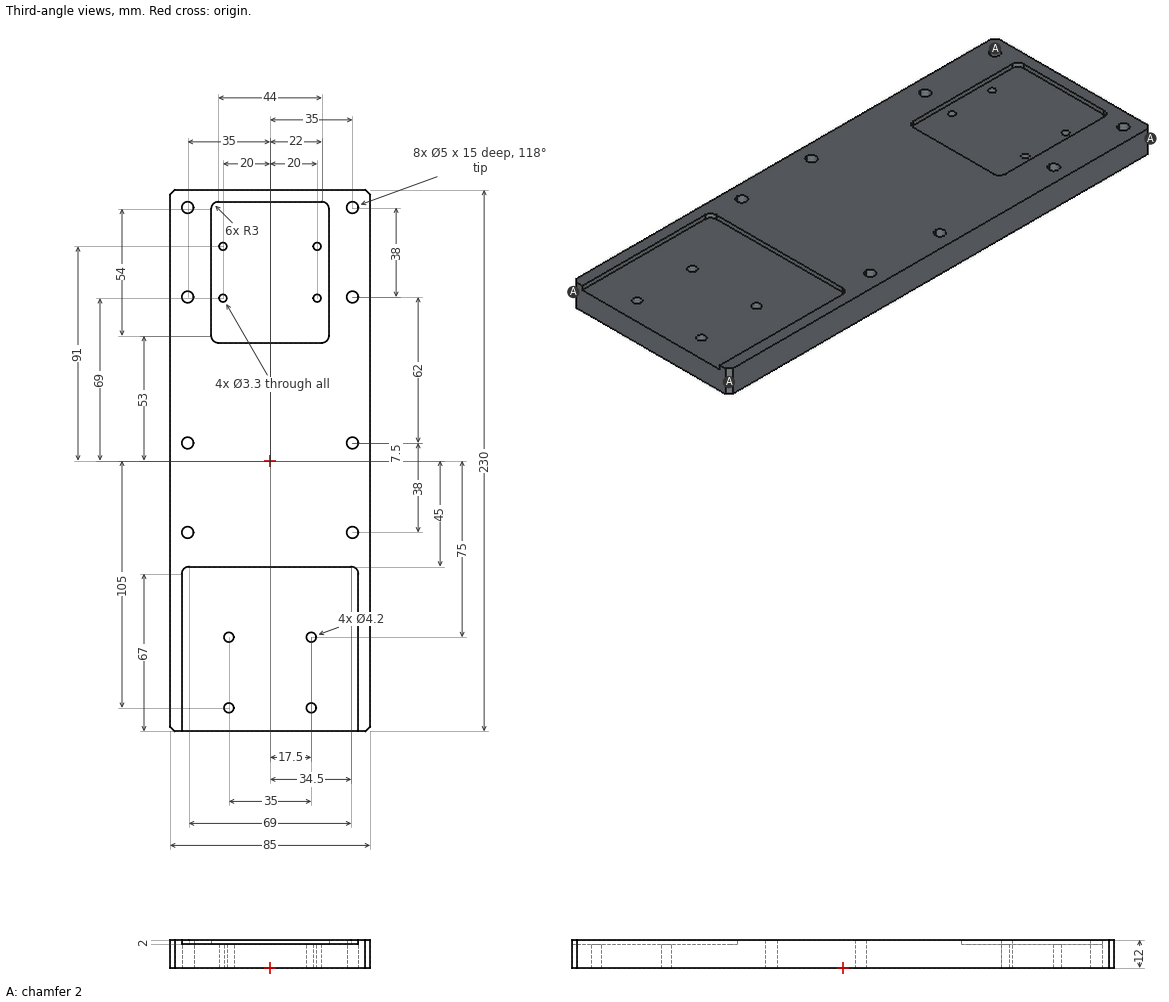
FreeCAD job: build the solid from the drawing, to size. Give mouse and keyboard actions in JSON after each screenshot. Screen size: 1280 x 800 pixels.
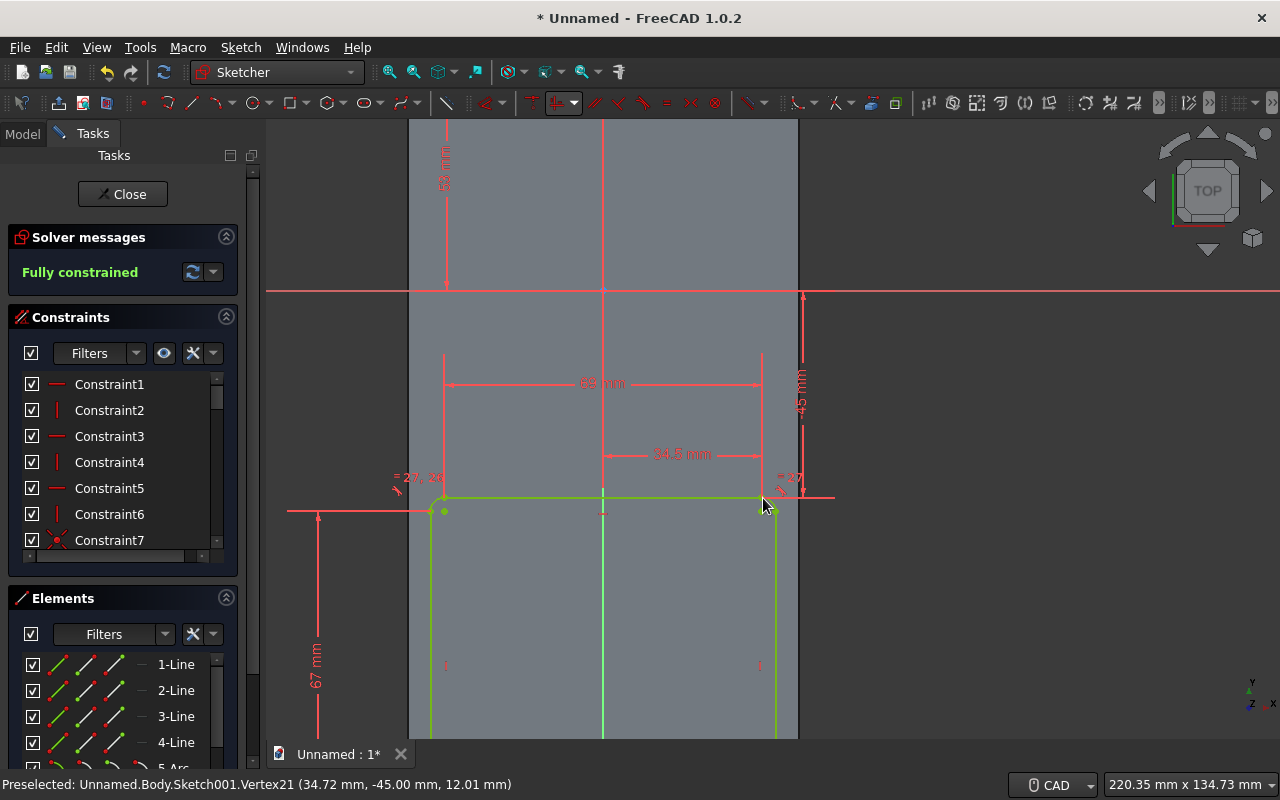
{"action": "left_click", "coordinate": [123, 194]}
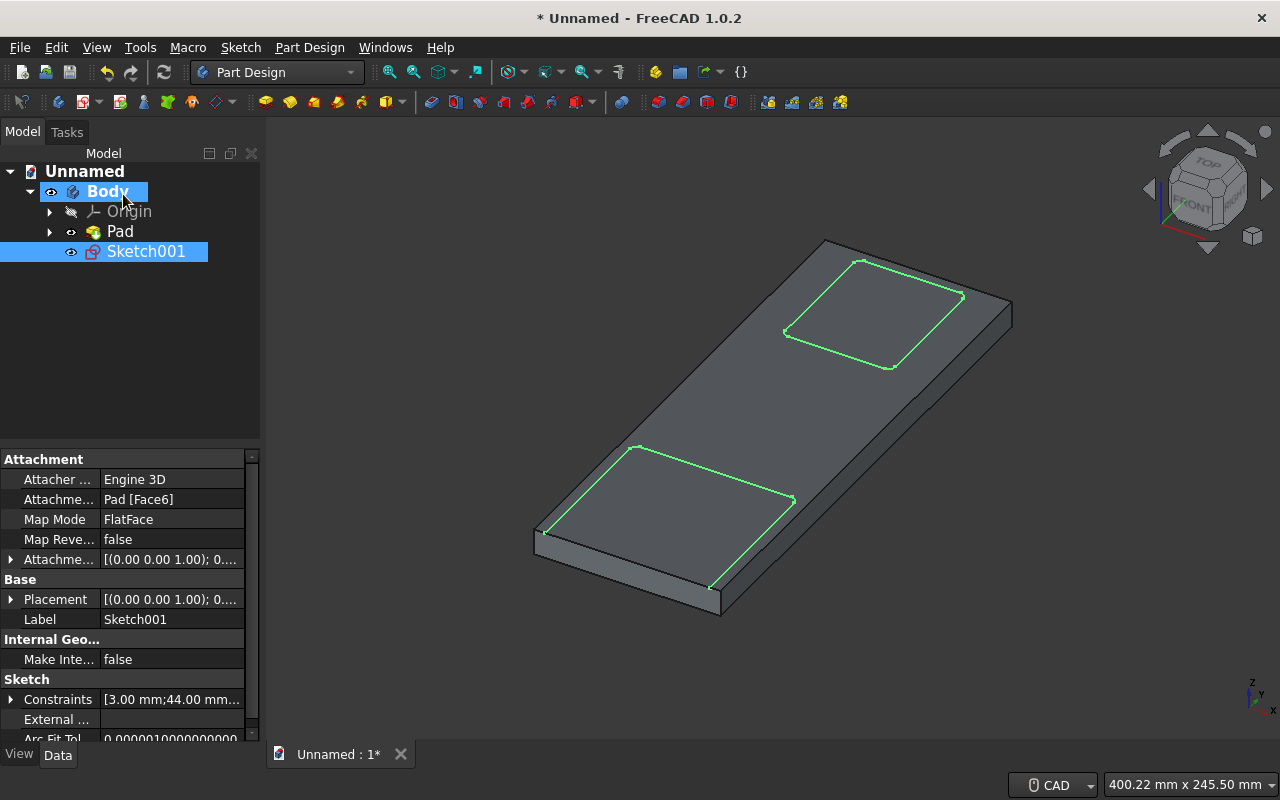
{"action": "left_click", "coordinate": [432, 102]}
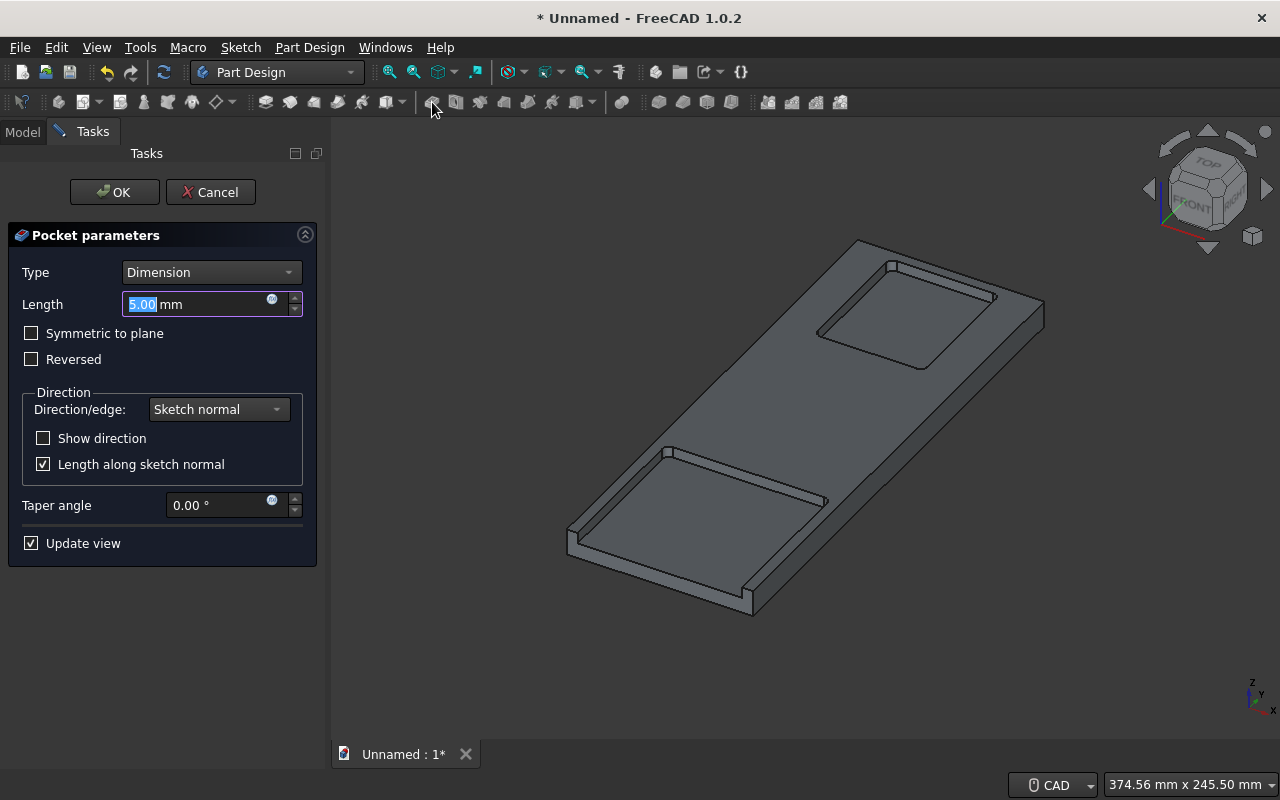
{"action": "type", "text": "2"}
{"action": "key", "text": "Tab"}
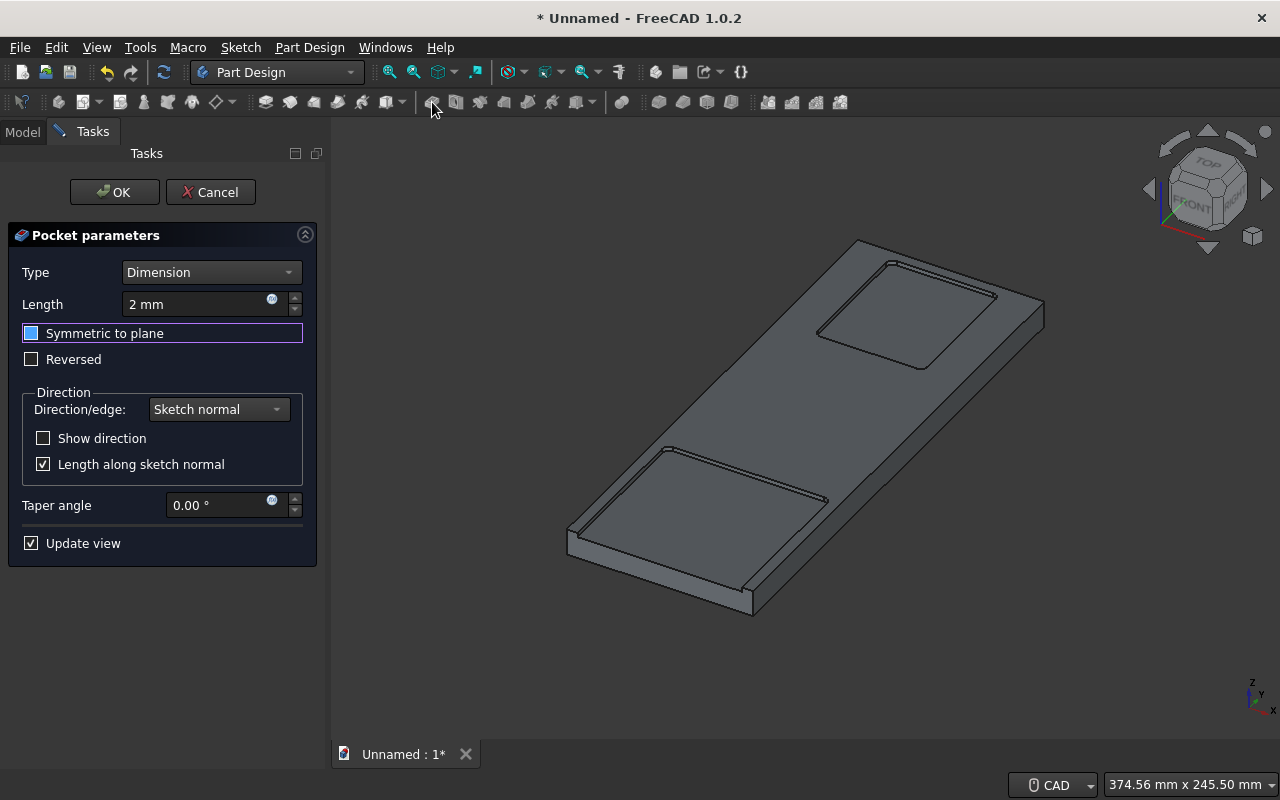
{"action": "left_click", "coordinate": [115, 192]}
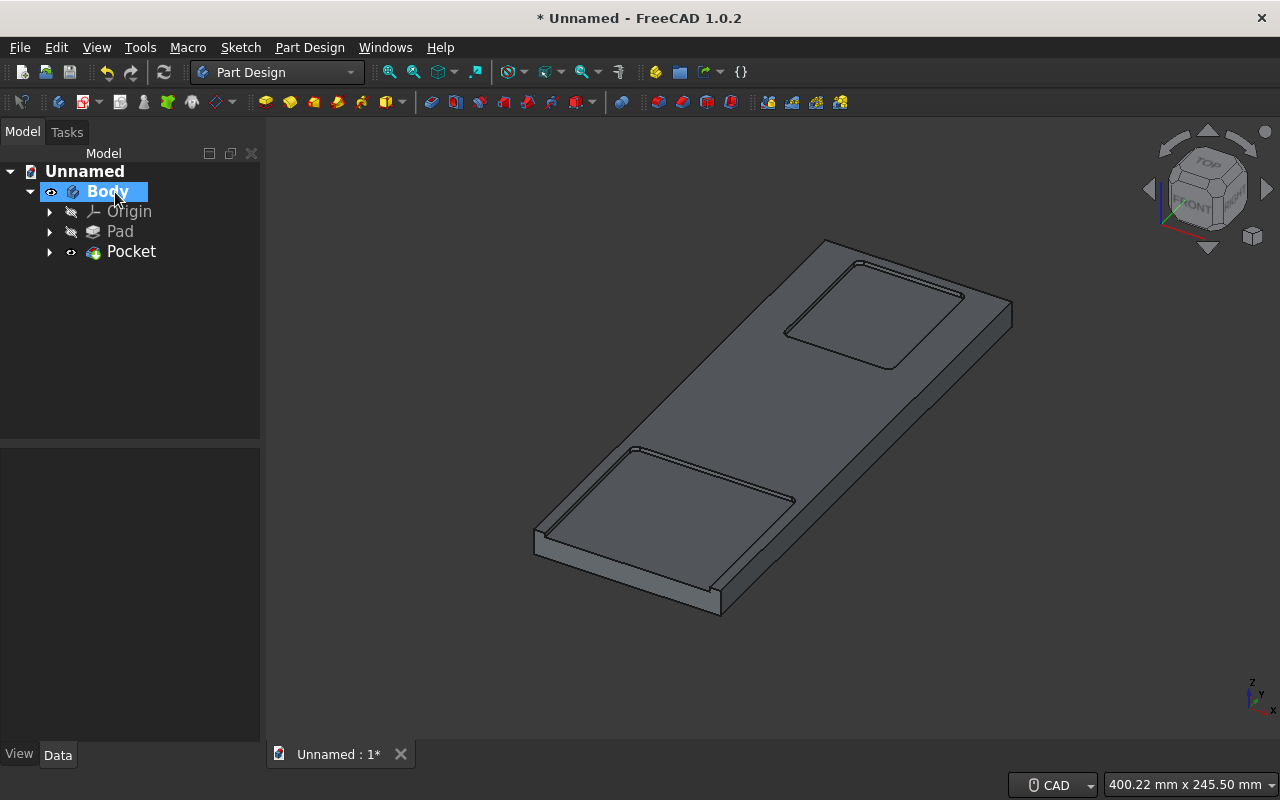
{"action": "left_click", "coordinate": [84, 102]}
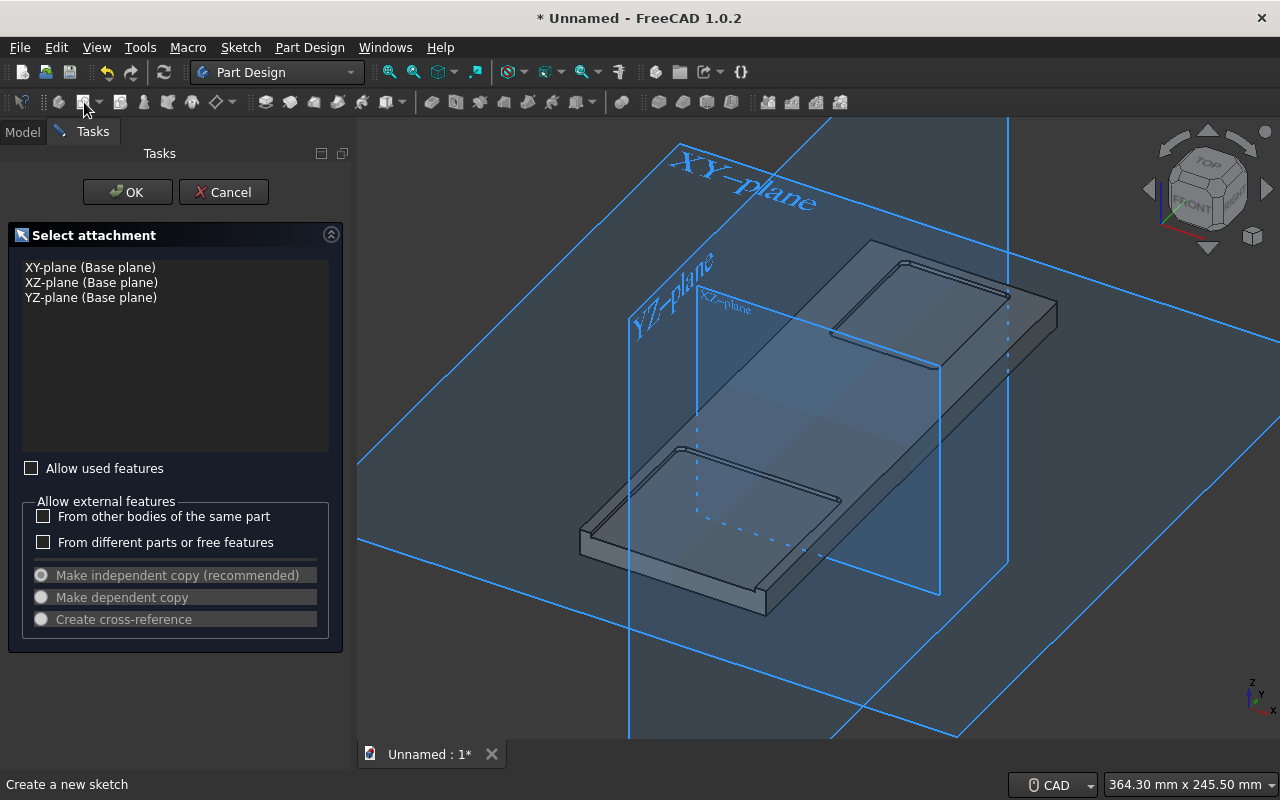
{"action": "left_click", "coordinate": [82, 268]}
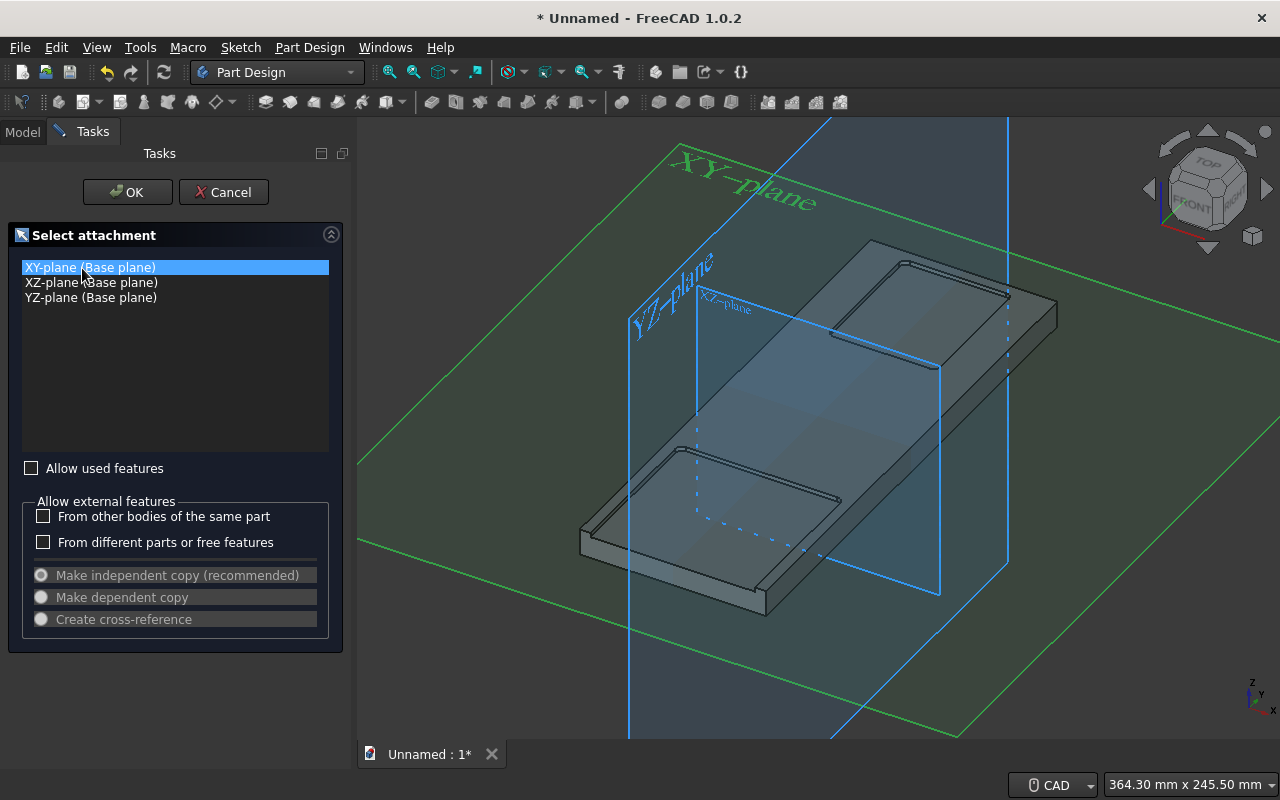
{"action": "left_click", "coordinate": [128, 192]}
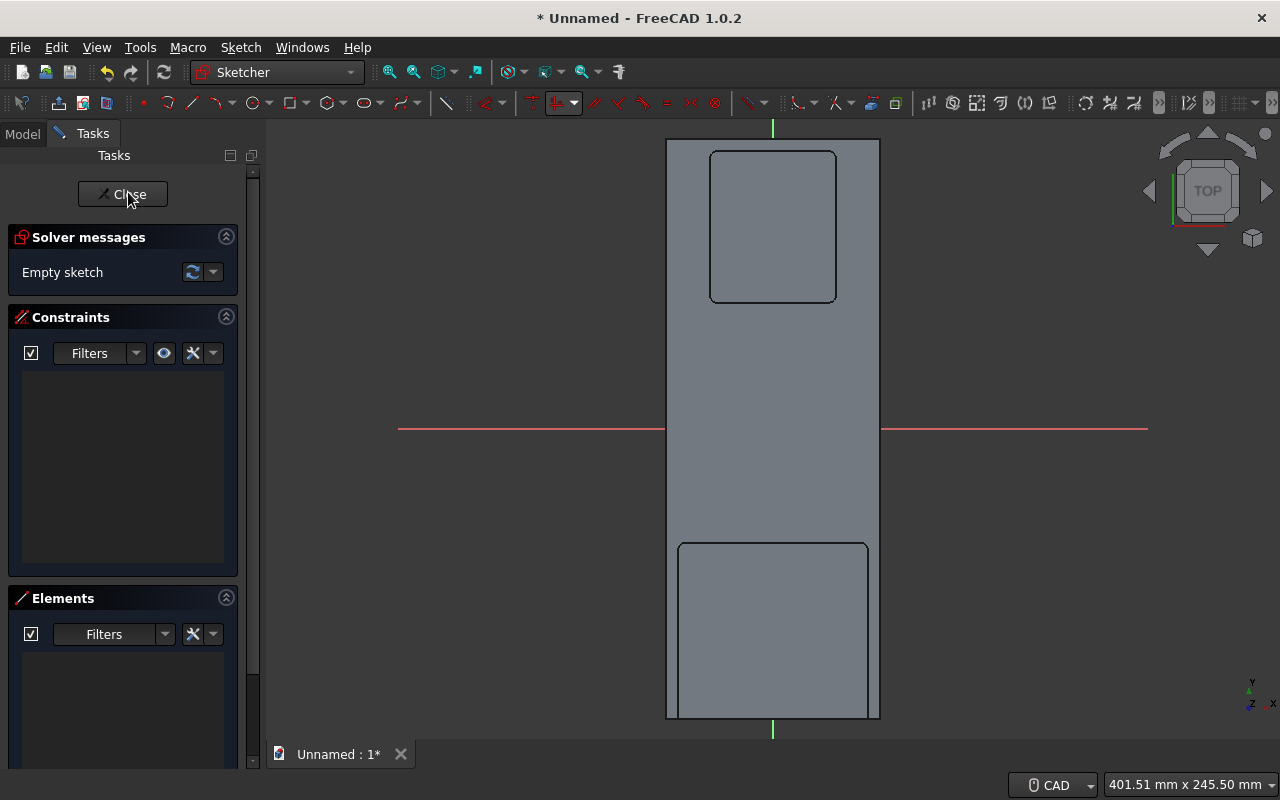
{"action": "left_click", "coordinate": [108, 104]}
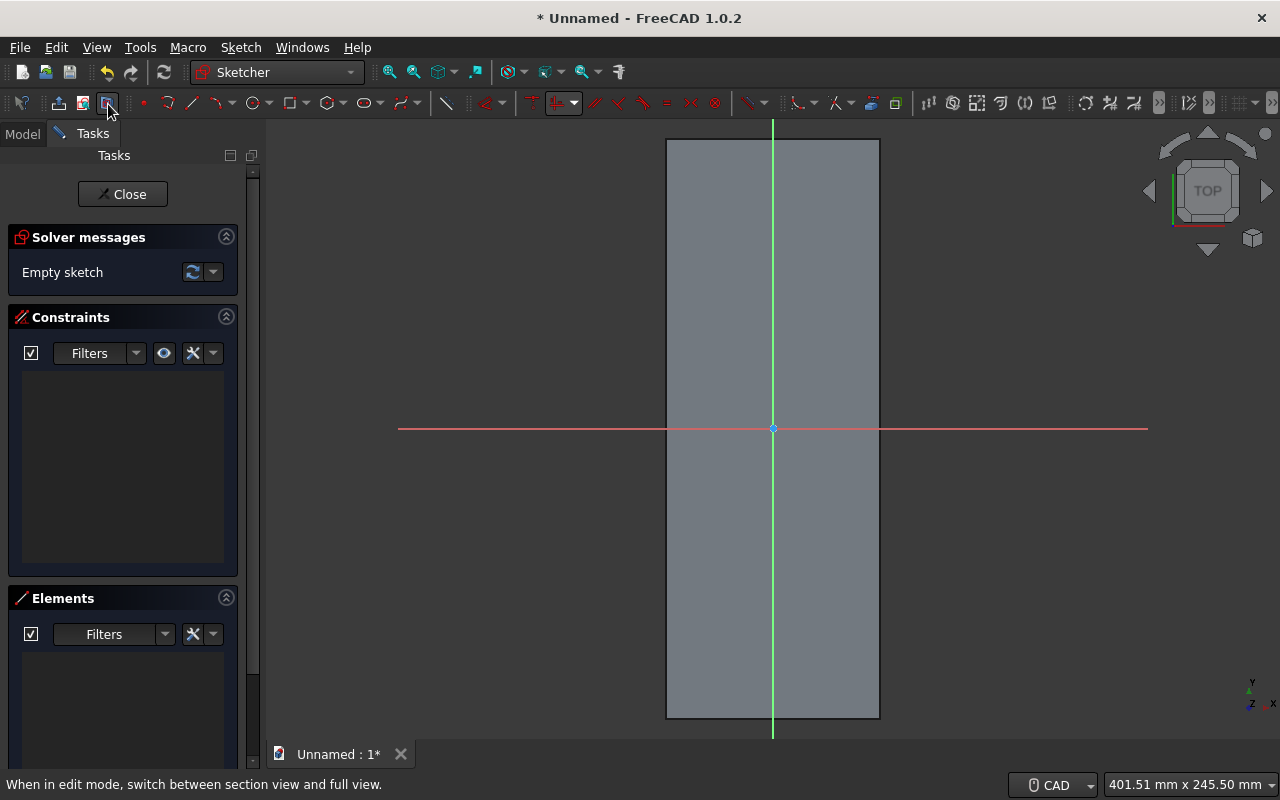
{"action": "scroll", "coordinate": [790, 711], "scroll_direction": "up", "scroll_amount": 8}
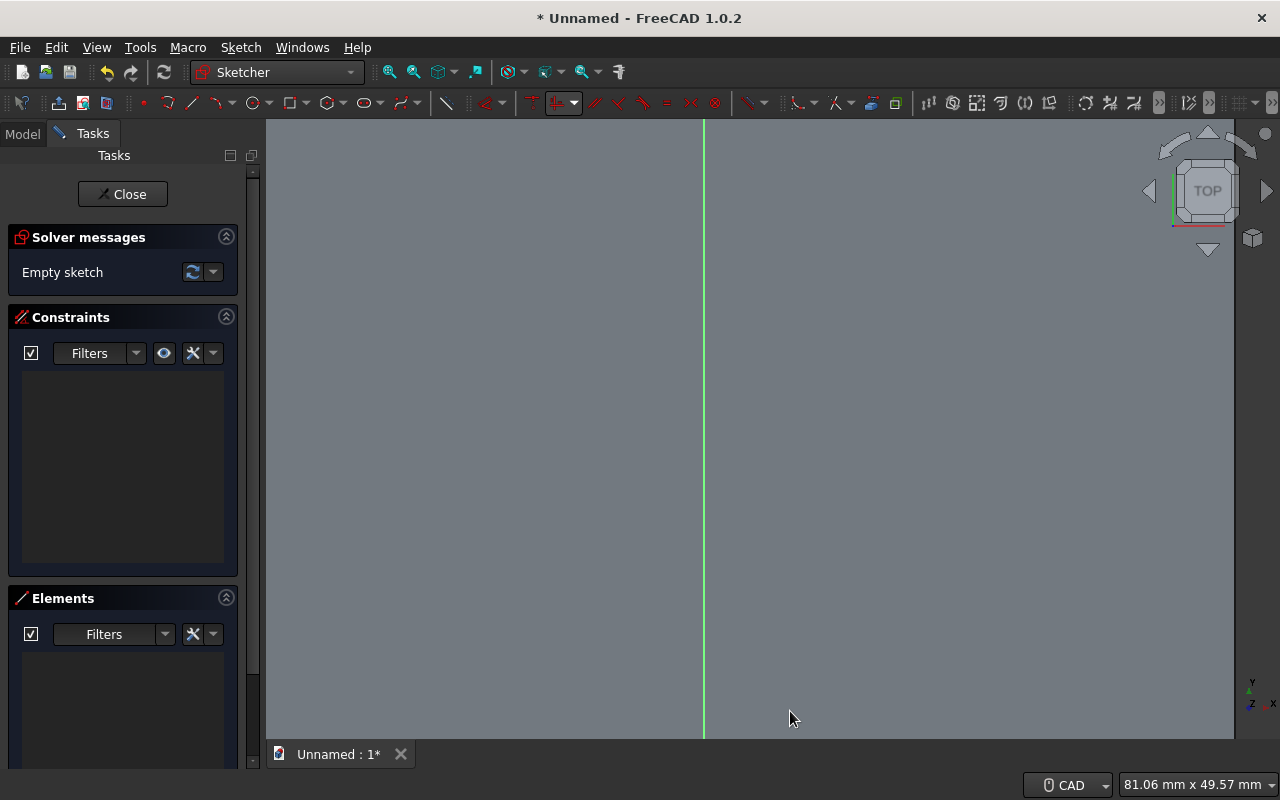
{"action": "key", "text": "g c"}